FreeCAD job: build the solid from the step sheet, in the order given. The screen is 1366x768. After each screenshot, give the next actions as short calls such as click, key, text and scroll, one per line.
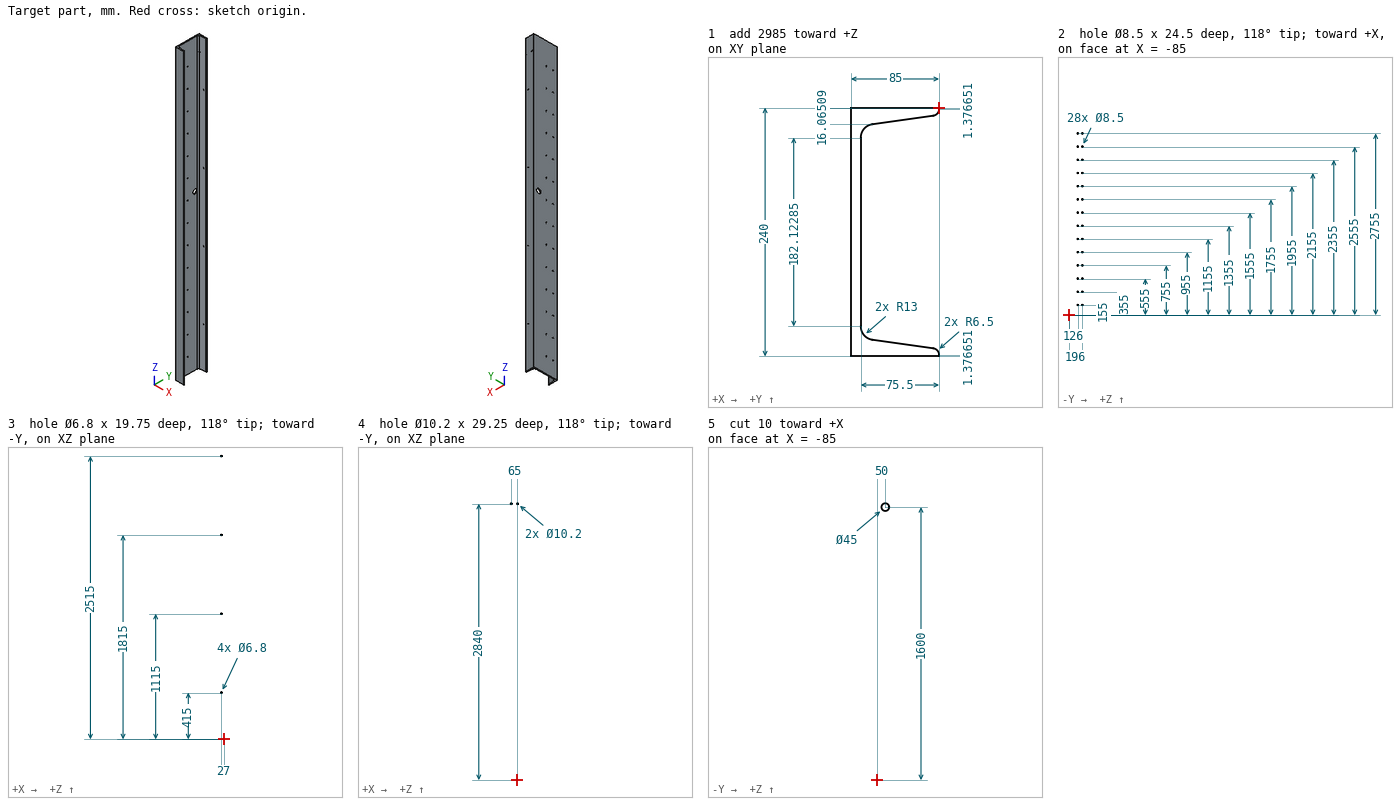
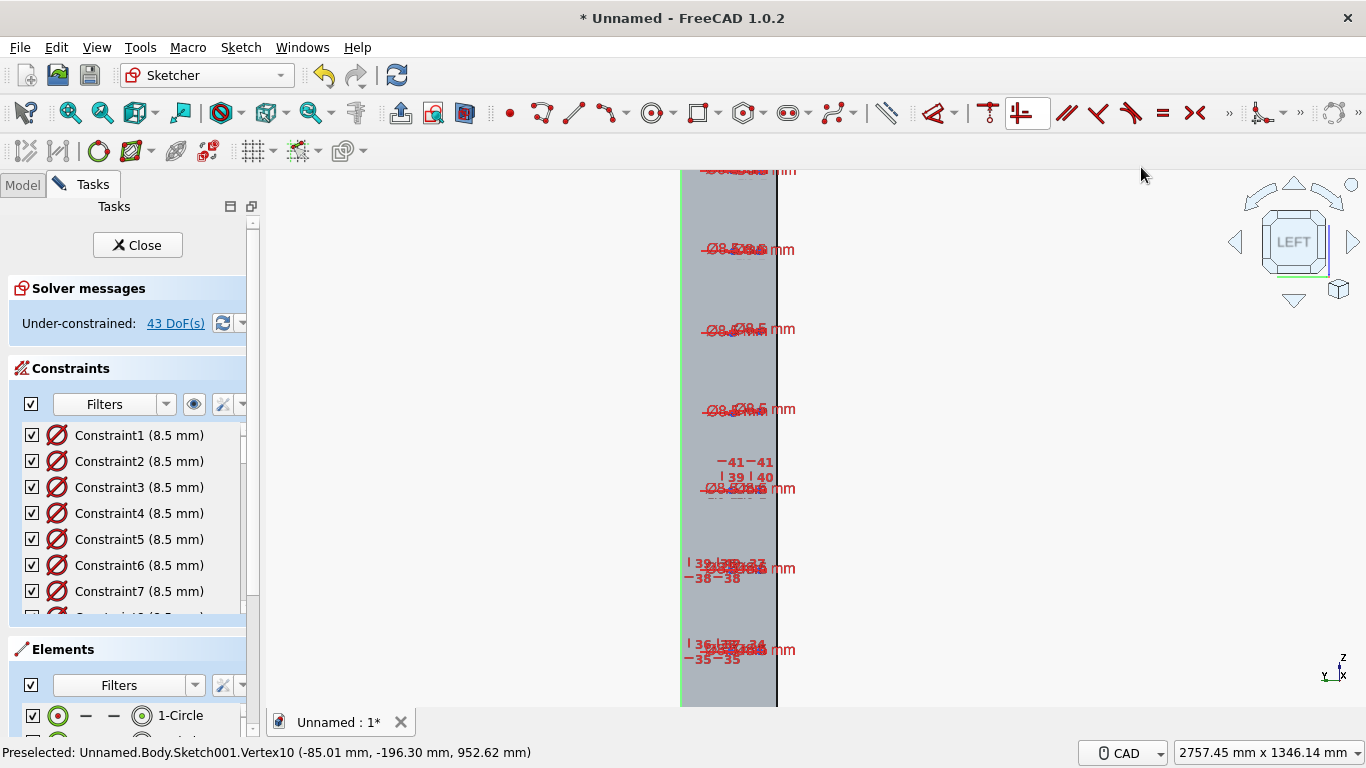
click(731, 491)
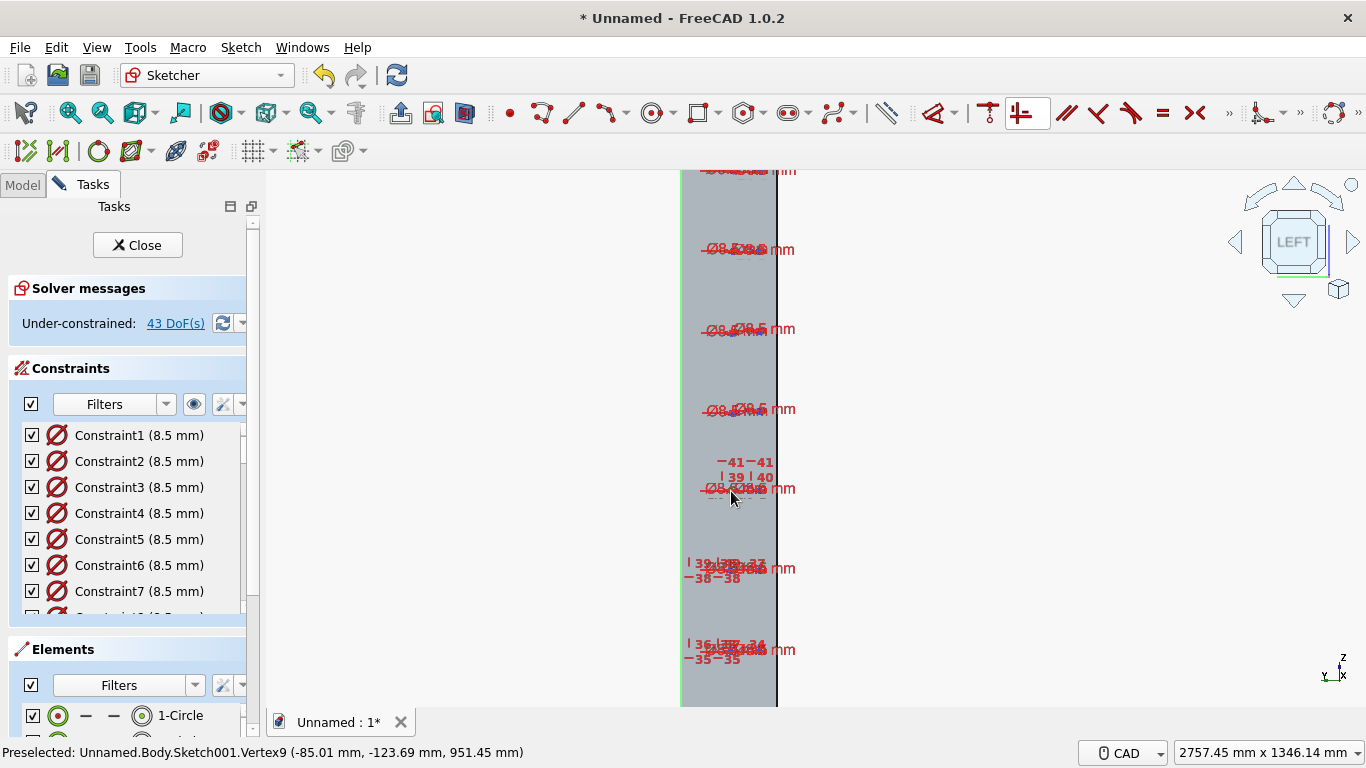
click(732, 413)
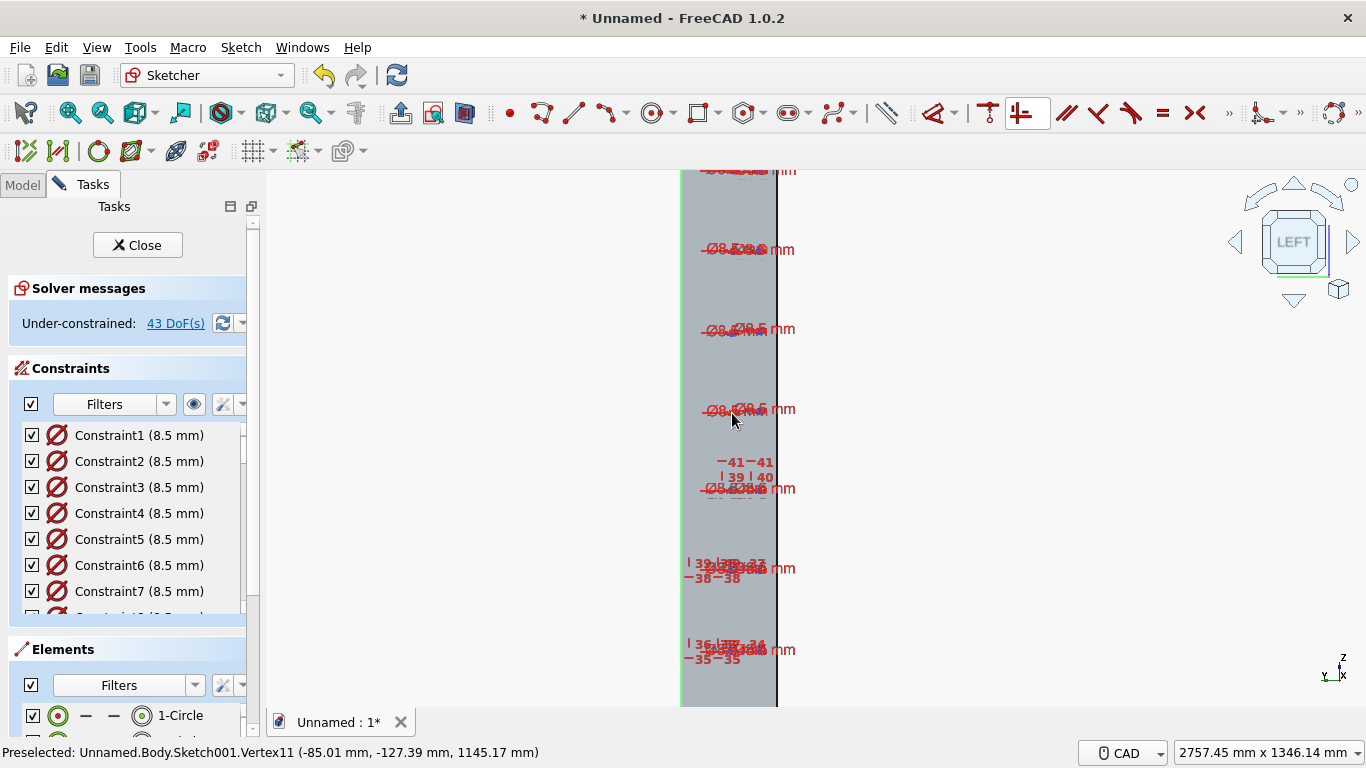
click(1044, 114)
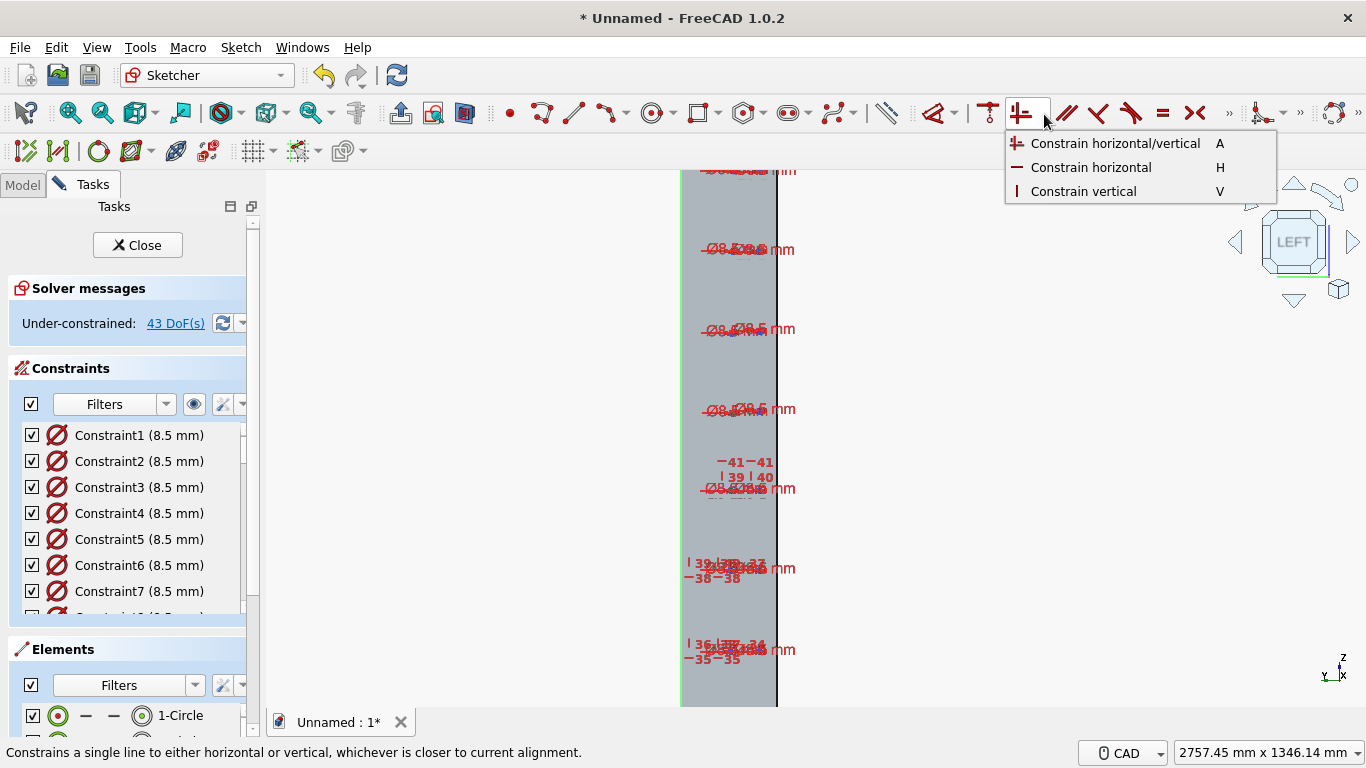
click(1141, 191)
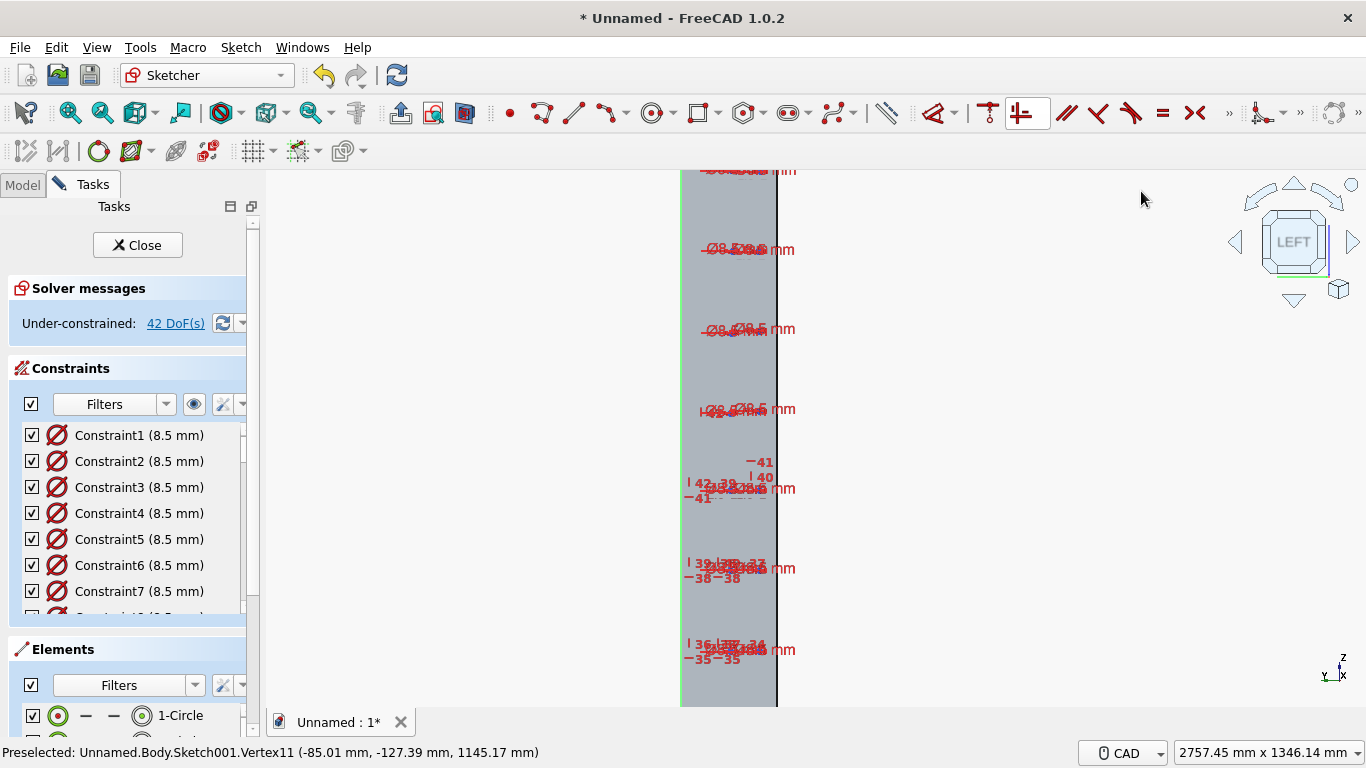
click(760, 491)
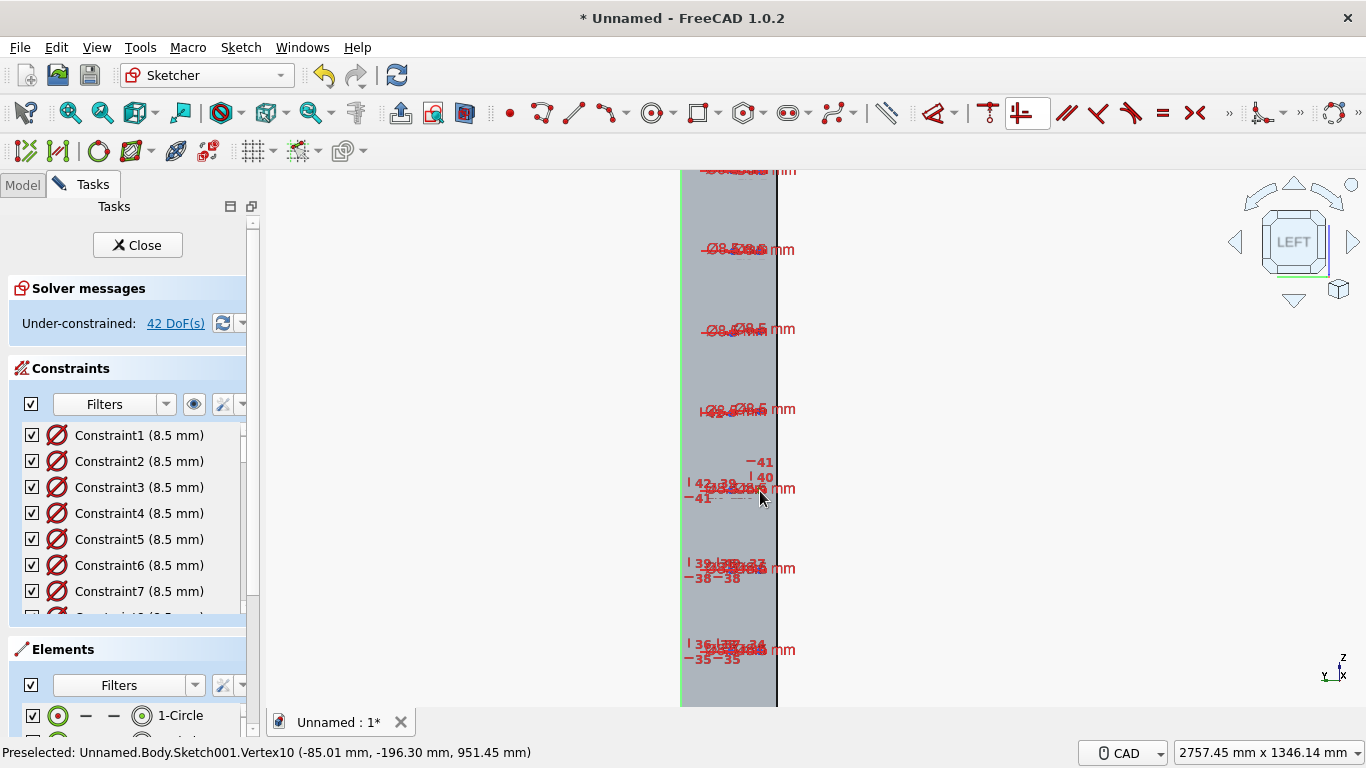
click(760, 411)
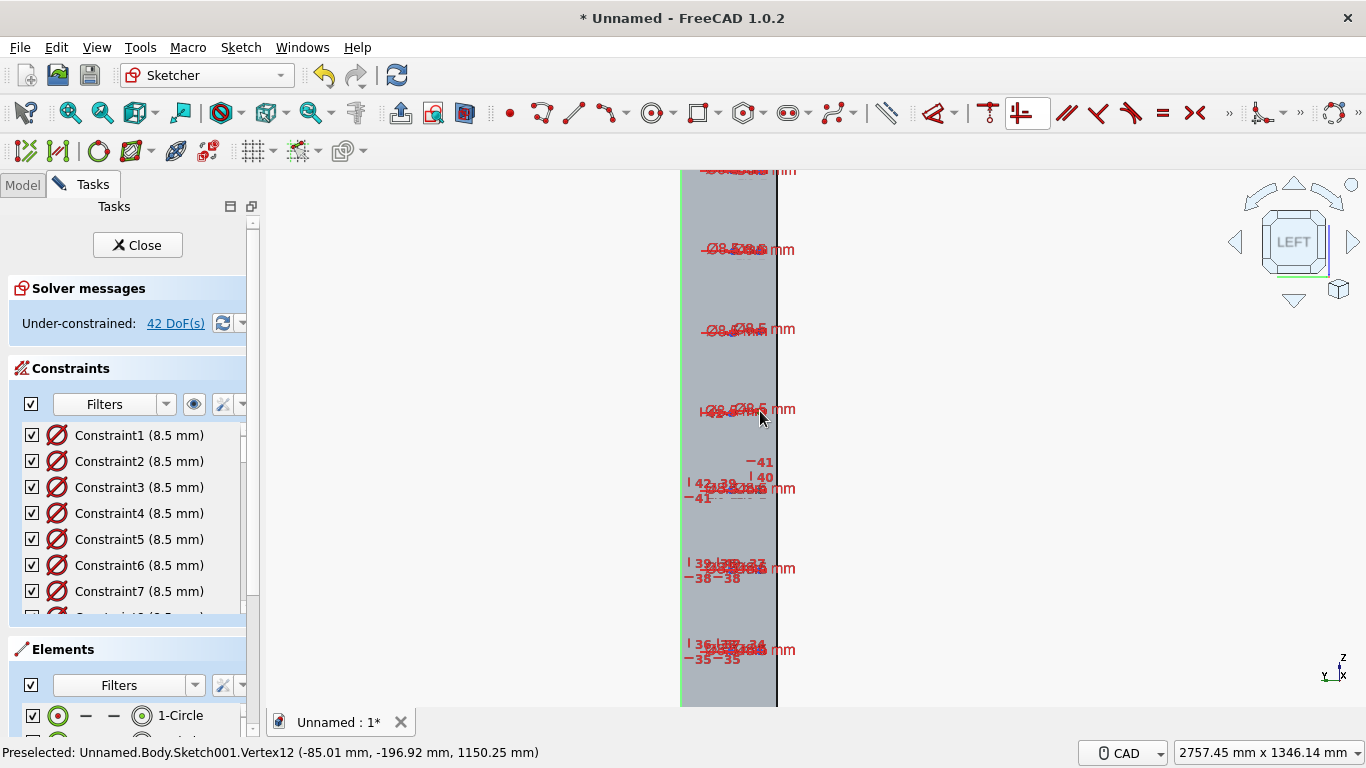
click(1044, 114)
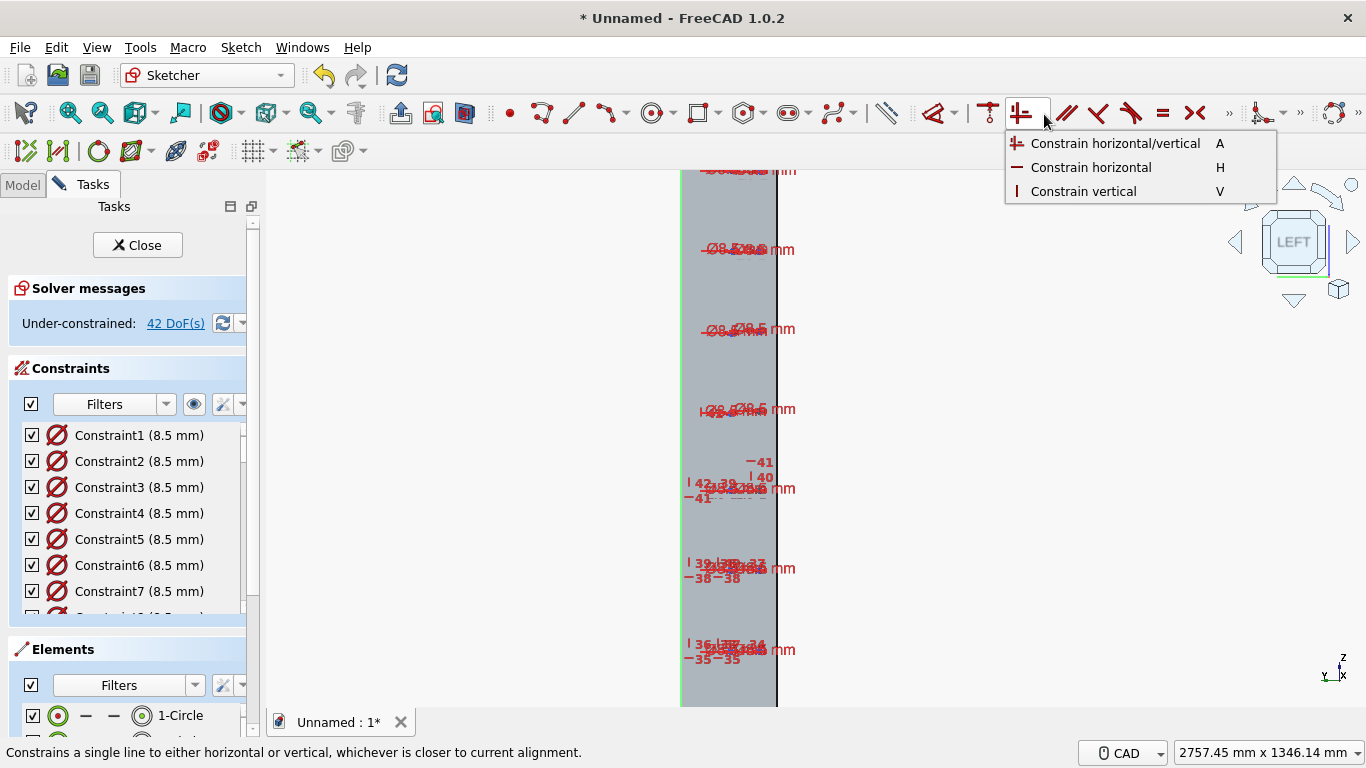
click(1141, 191)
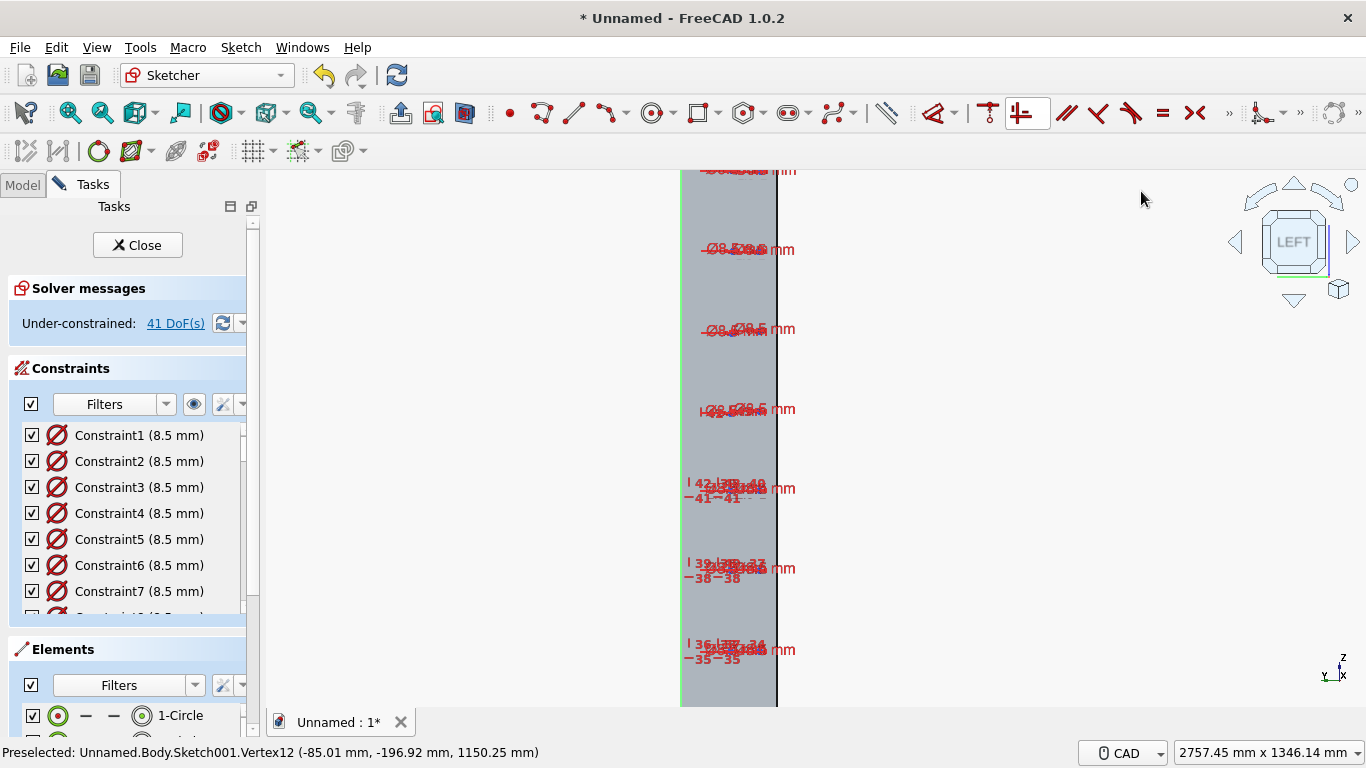
scroll(731, 413, up, 4)